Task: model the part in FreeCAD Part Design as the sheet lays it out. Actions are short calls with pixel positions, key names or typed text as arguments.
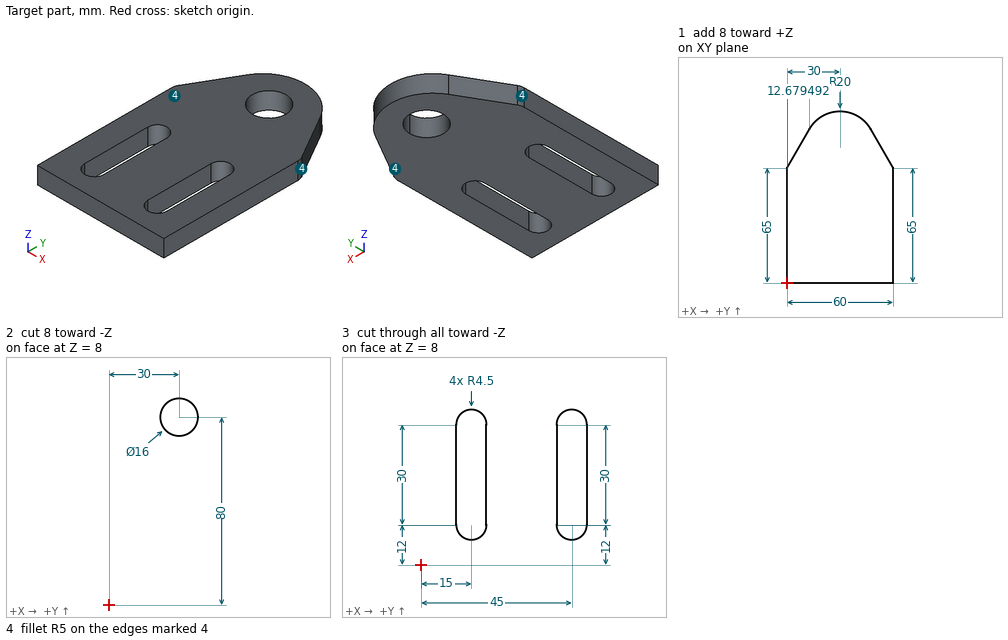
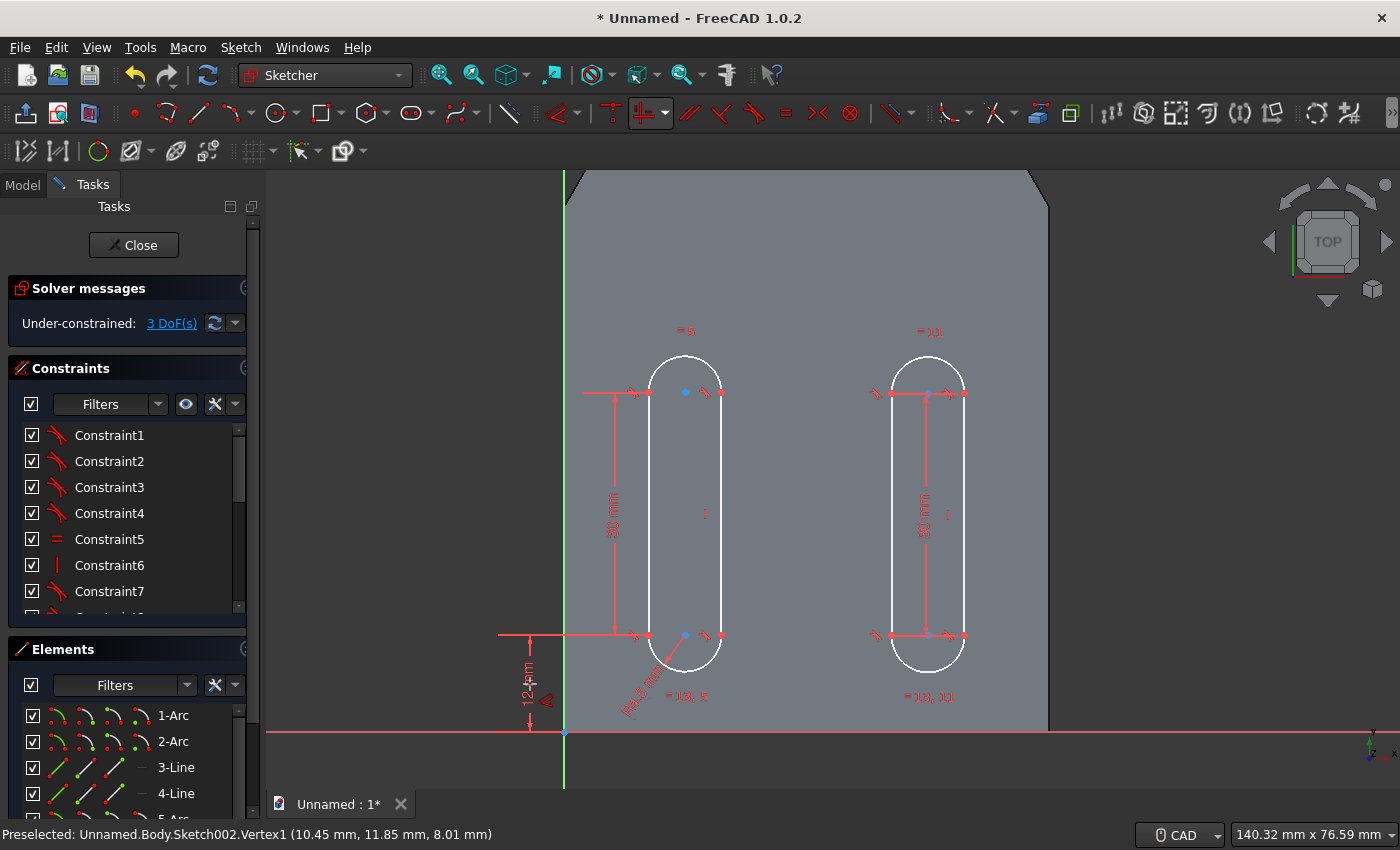
click(892, 636)
click(530, 662)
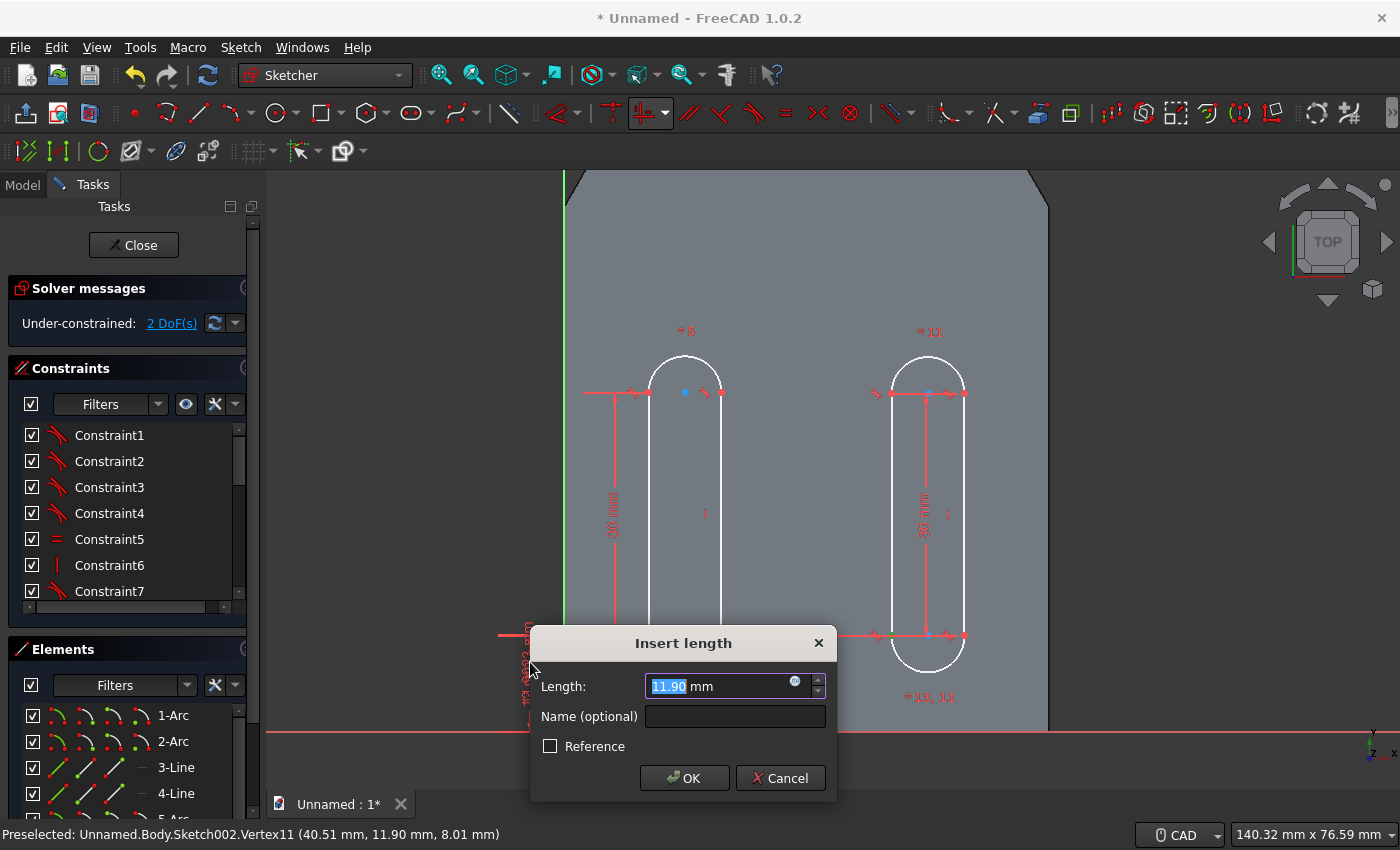
text(12)
key(Return)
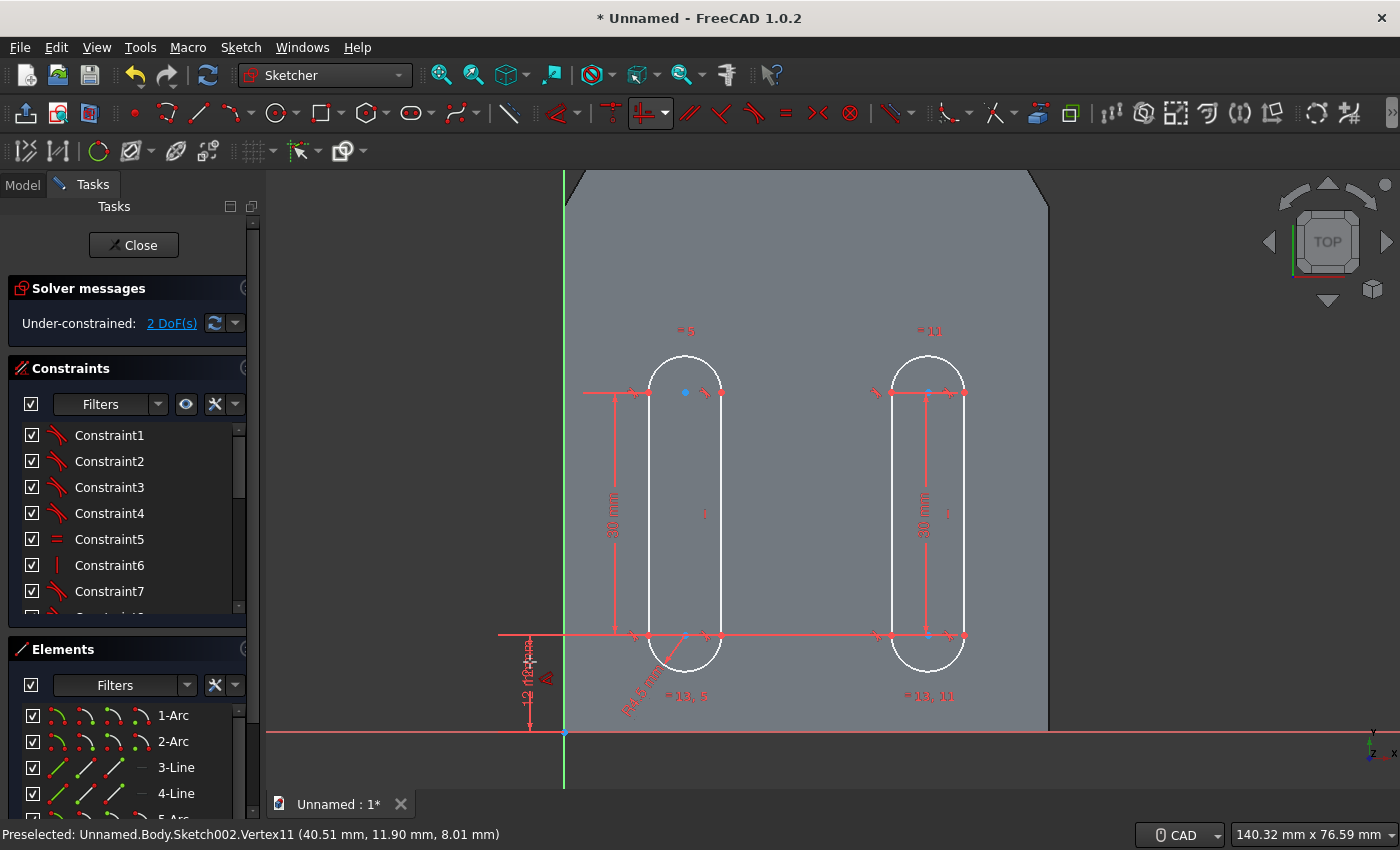
click(685, 635)
click(625, 601)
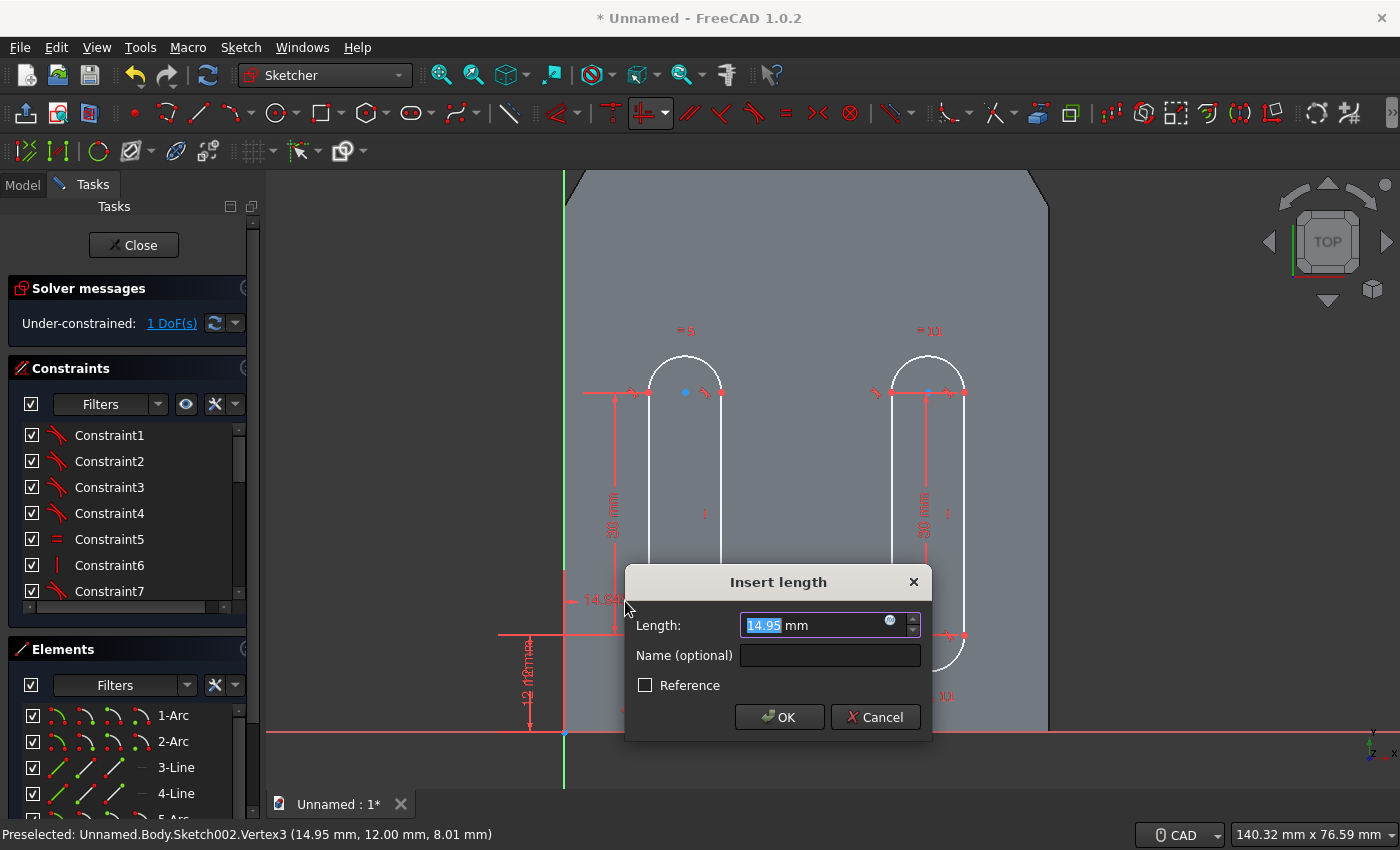
text(15)
key(Return)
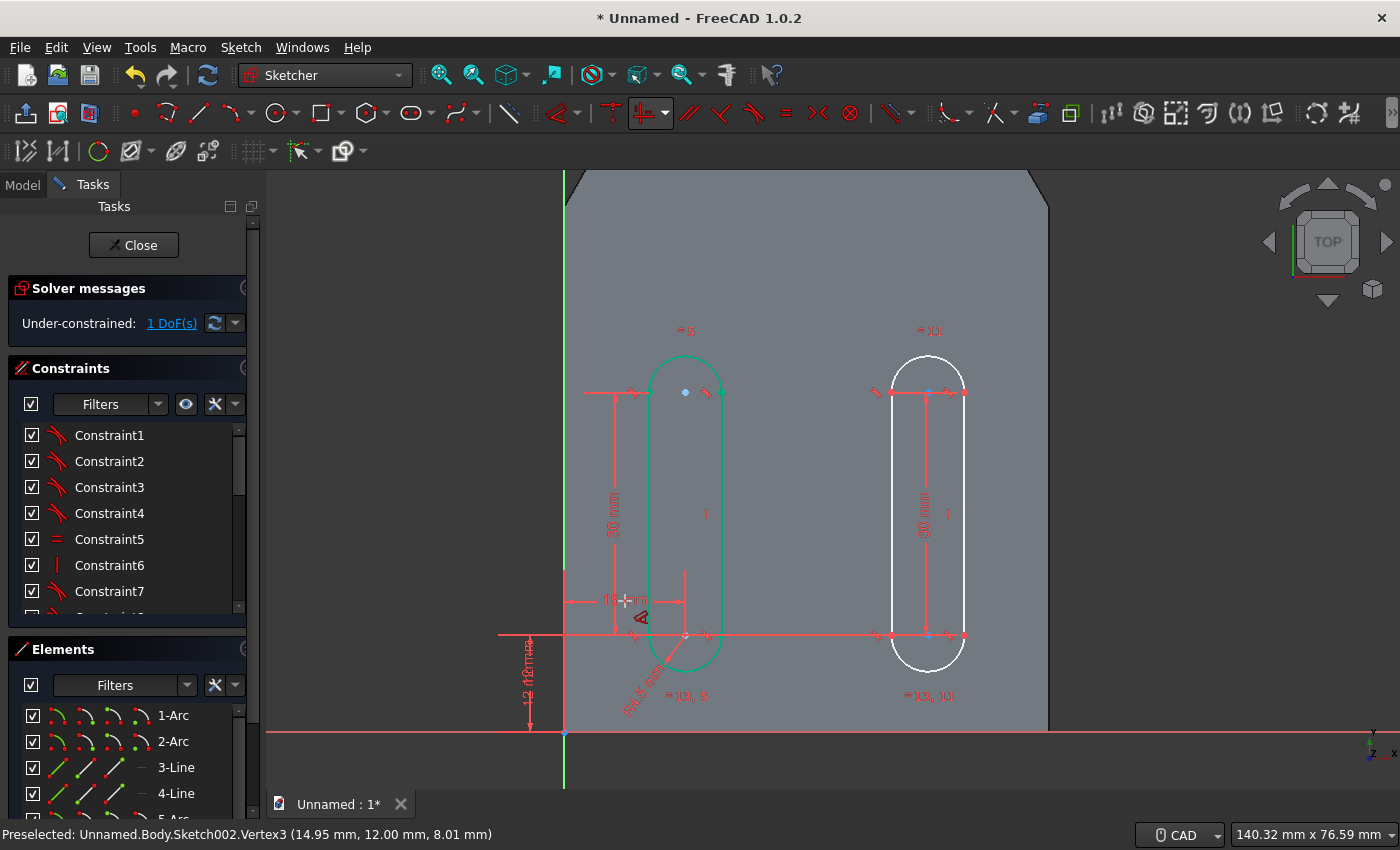
click(928, 635)
click(746, 601)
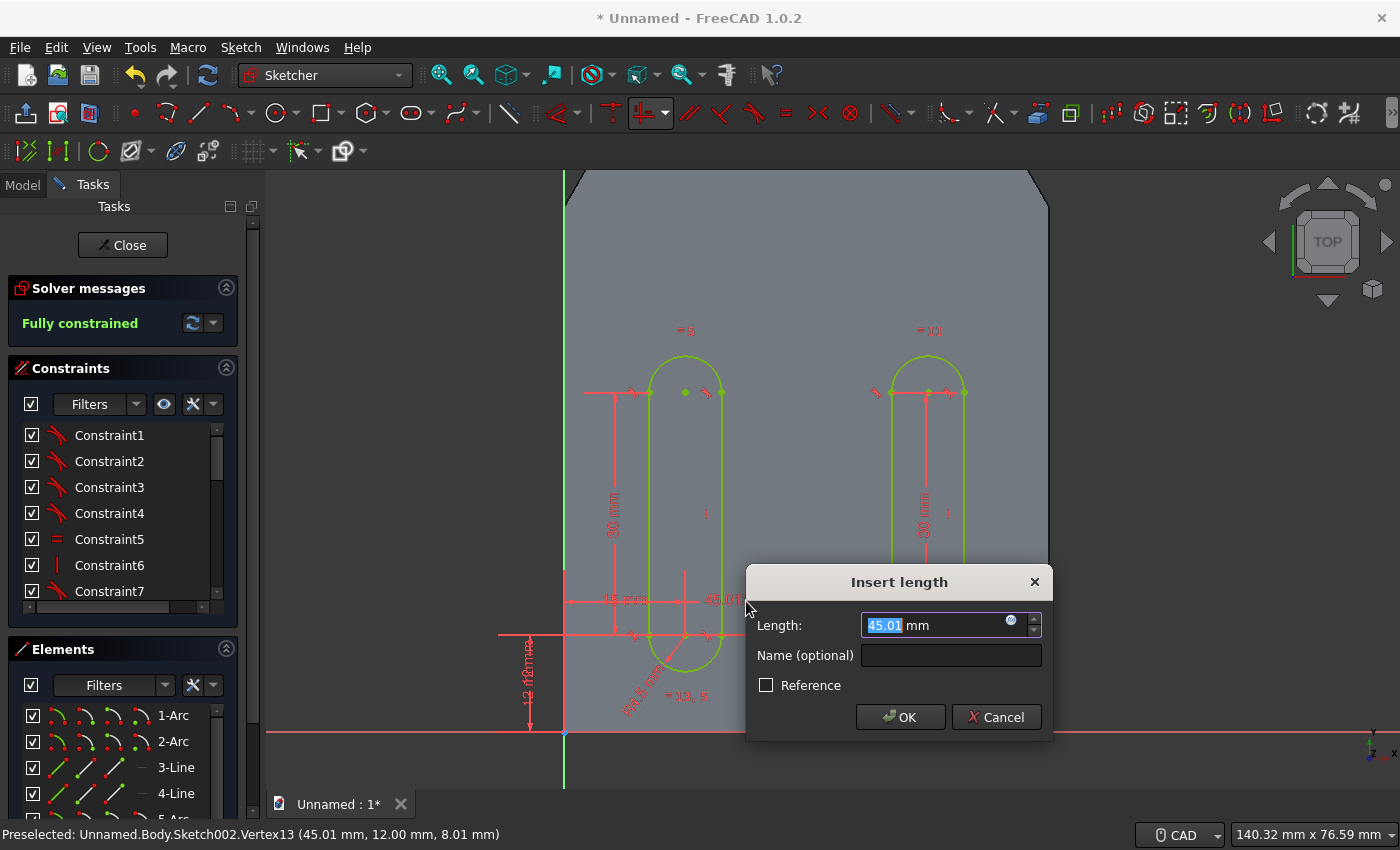
text(45)
key(Return)
key(Escape)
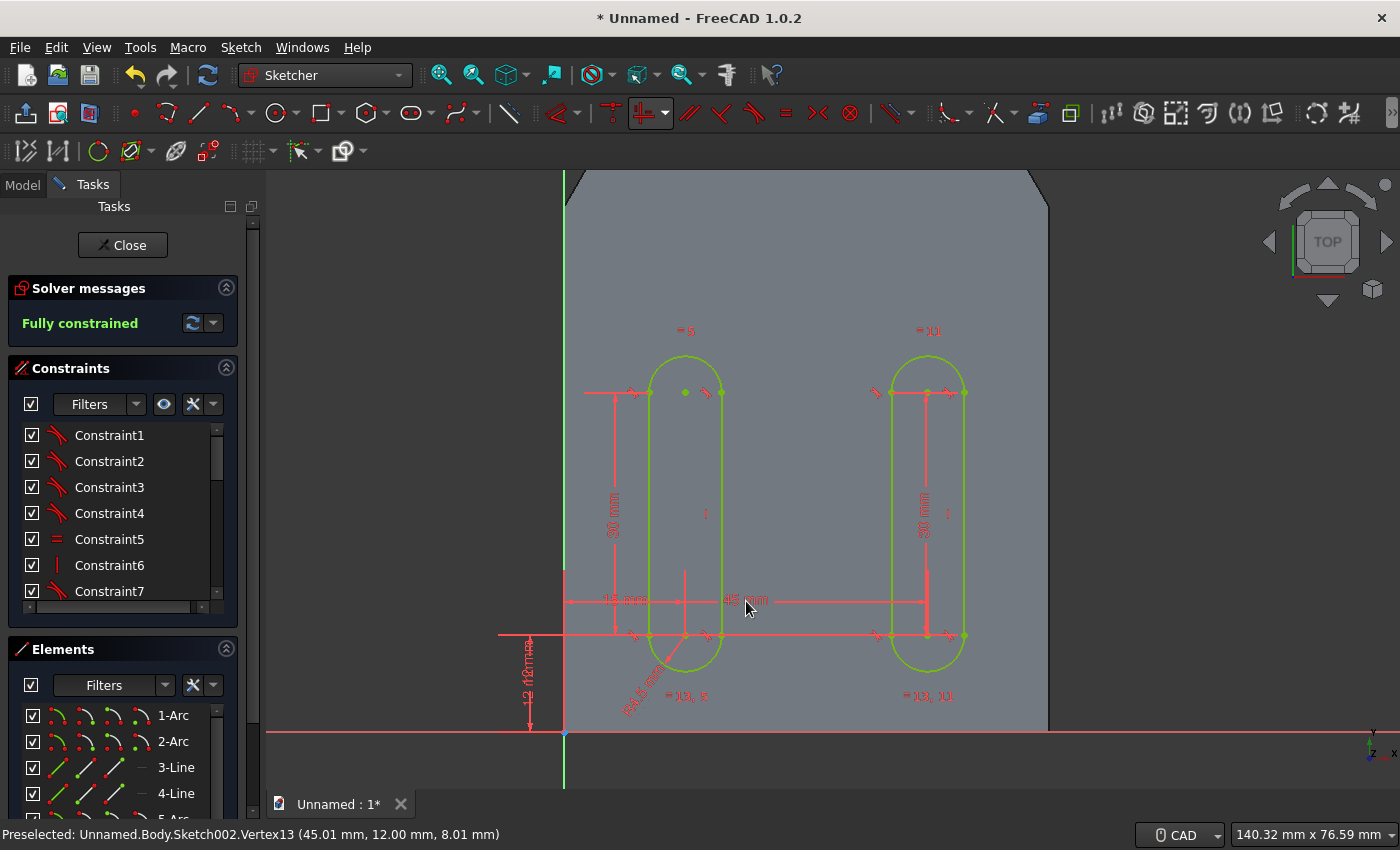
click(123, 245)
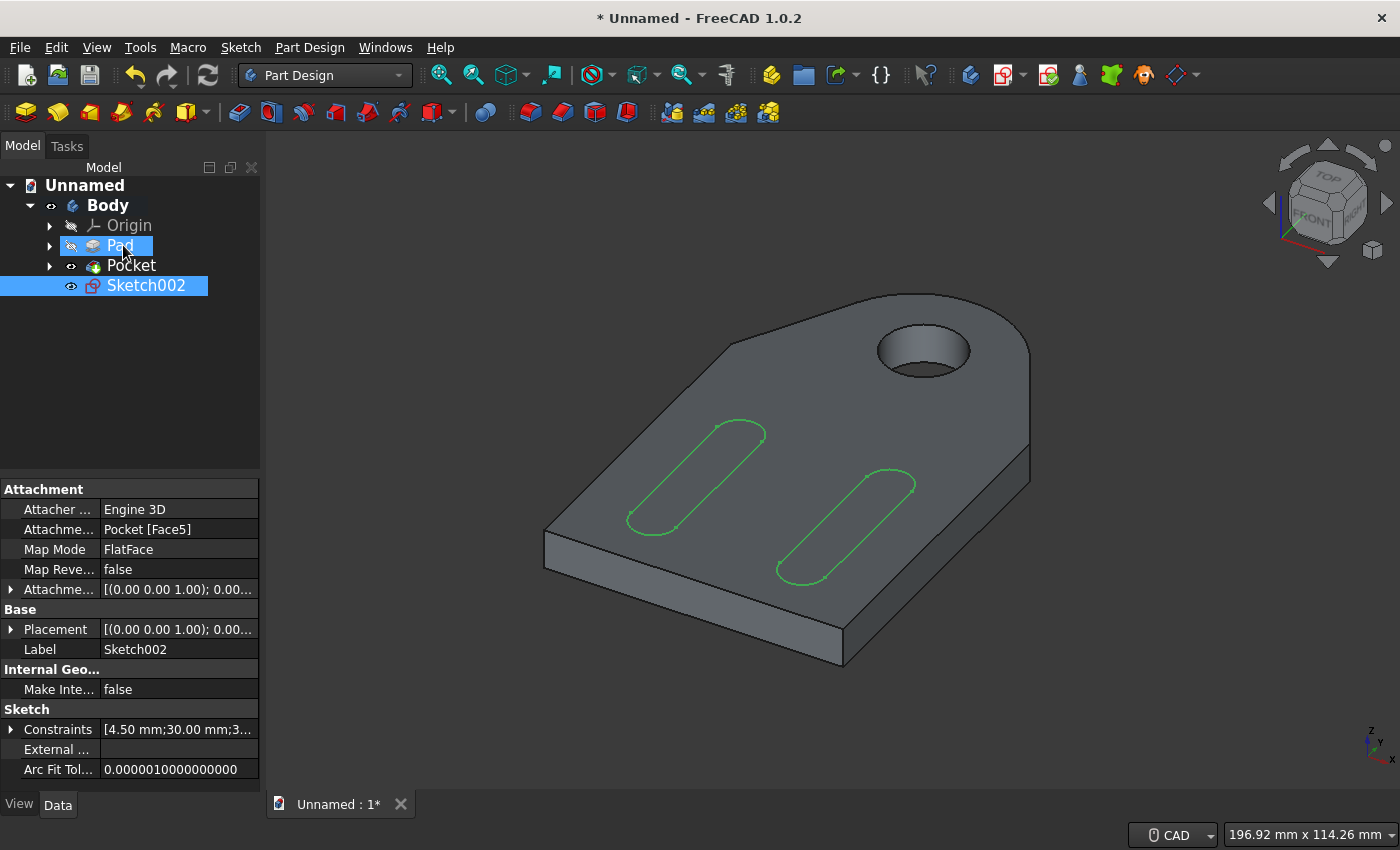
click(240, 112)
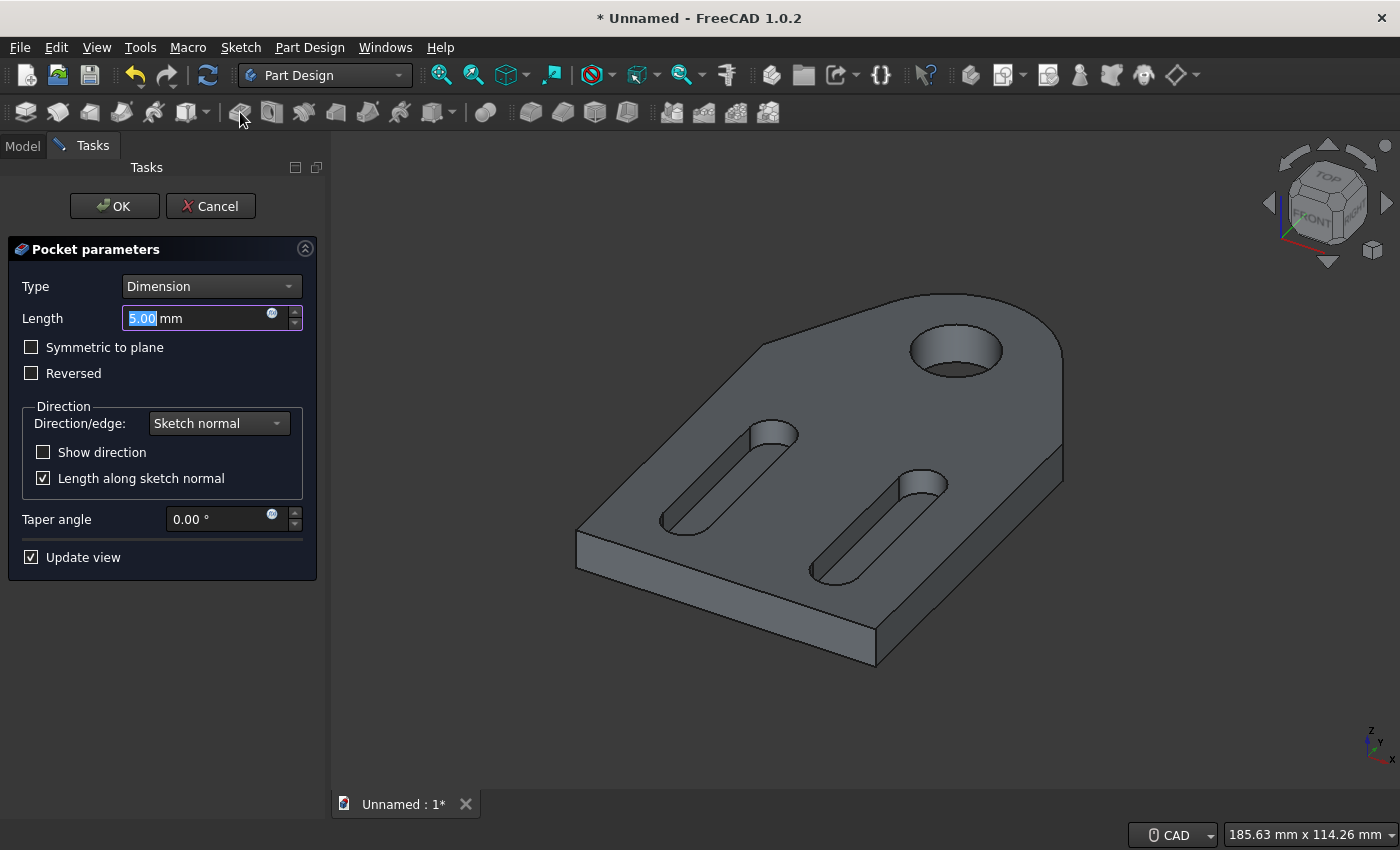
click(212, 286)